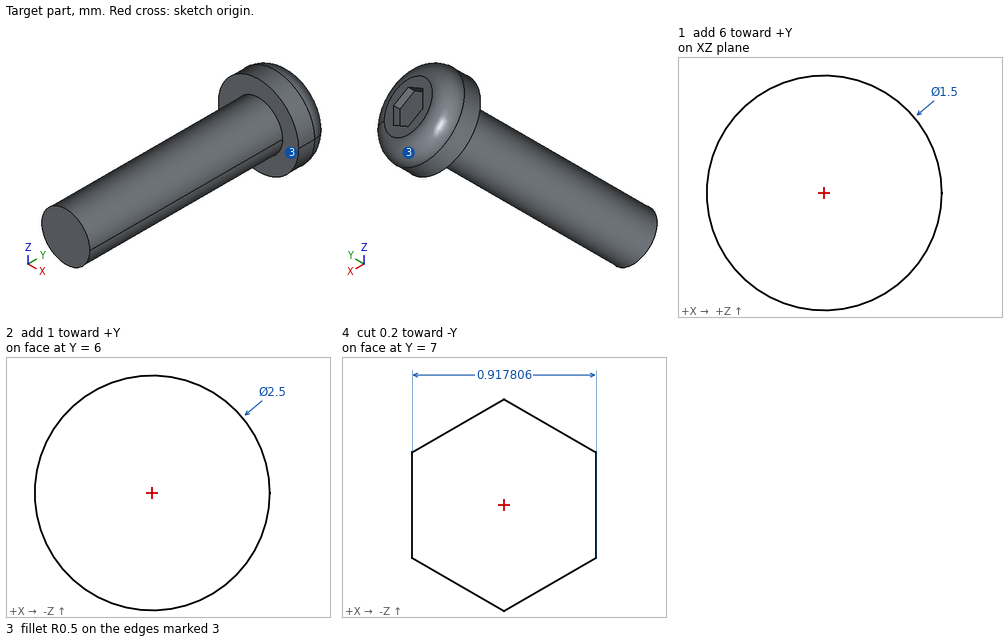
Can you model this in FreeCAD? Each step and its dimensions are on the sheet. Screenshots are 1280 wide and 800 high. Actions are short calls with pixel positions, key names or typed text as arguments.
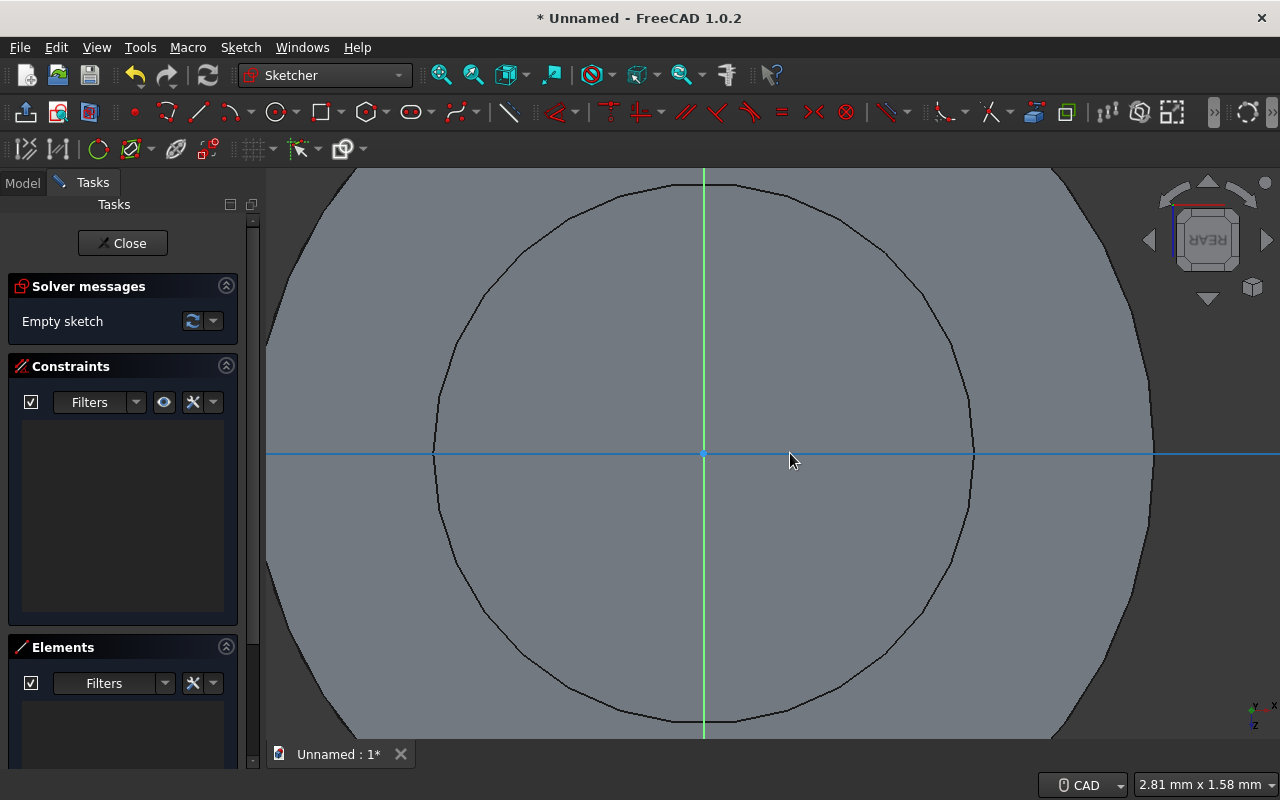
click(366, 112)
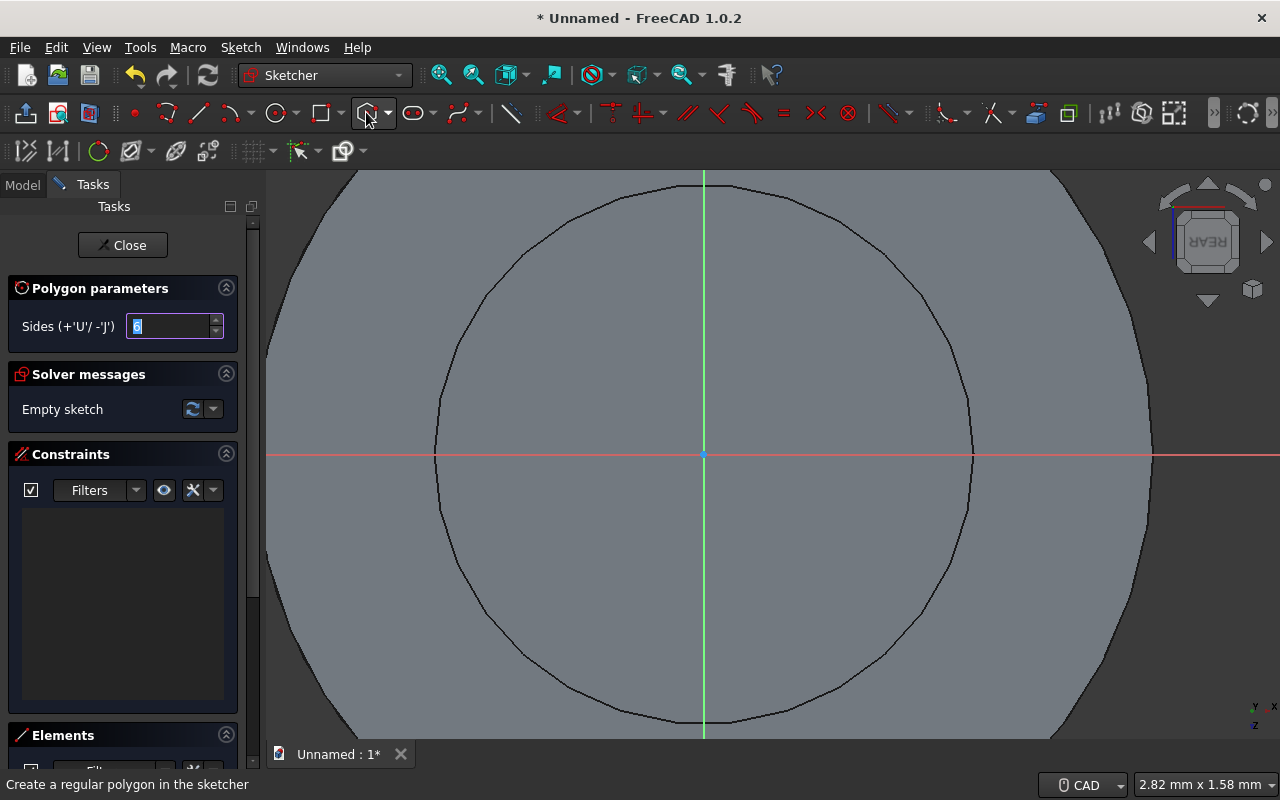
click(704, 454)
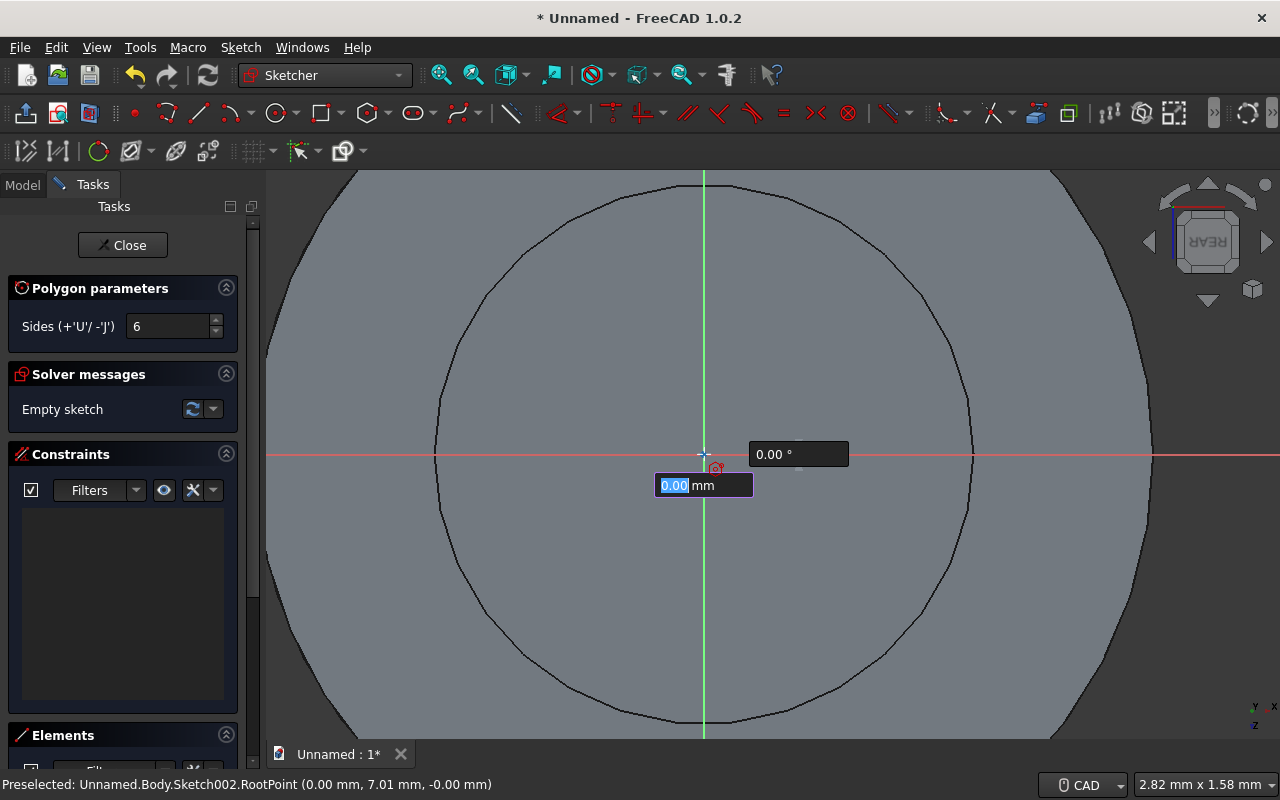
click(704, 264)
key(Escape)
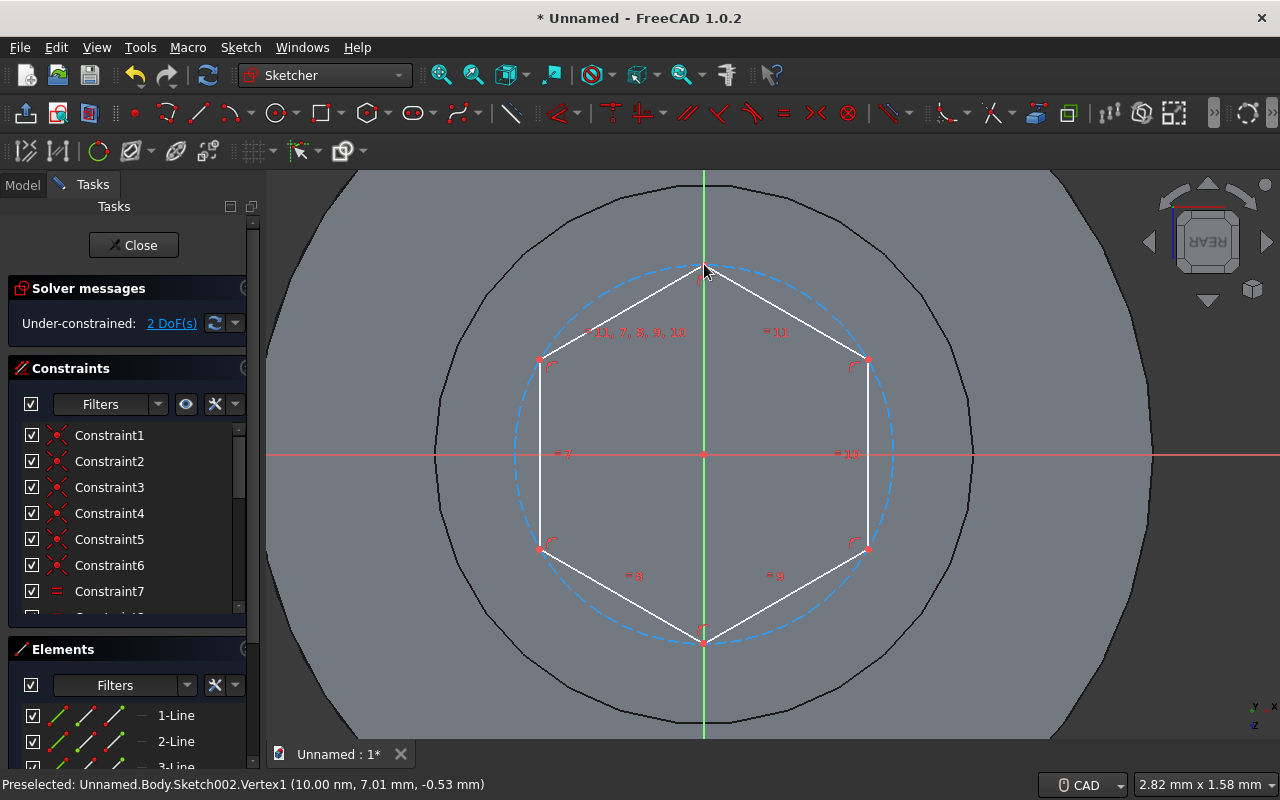
click(540, 417)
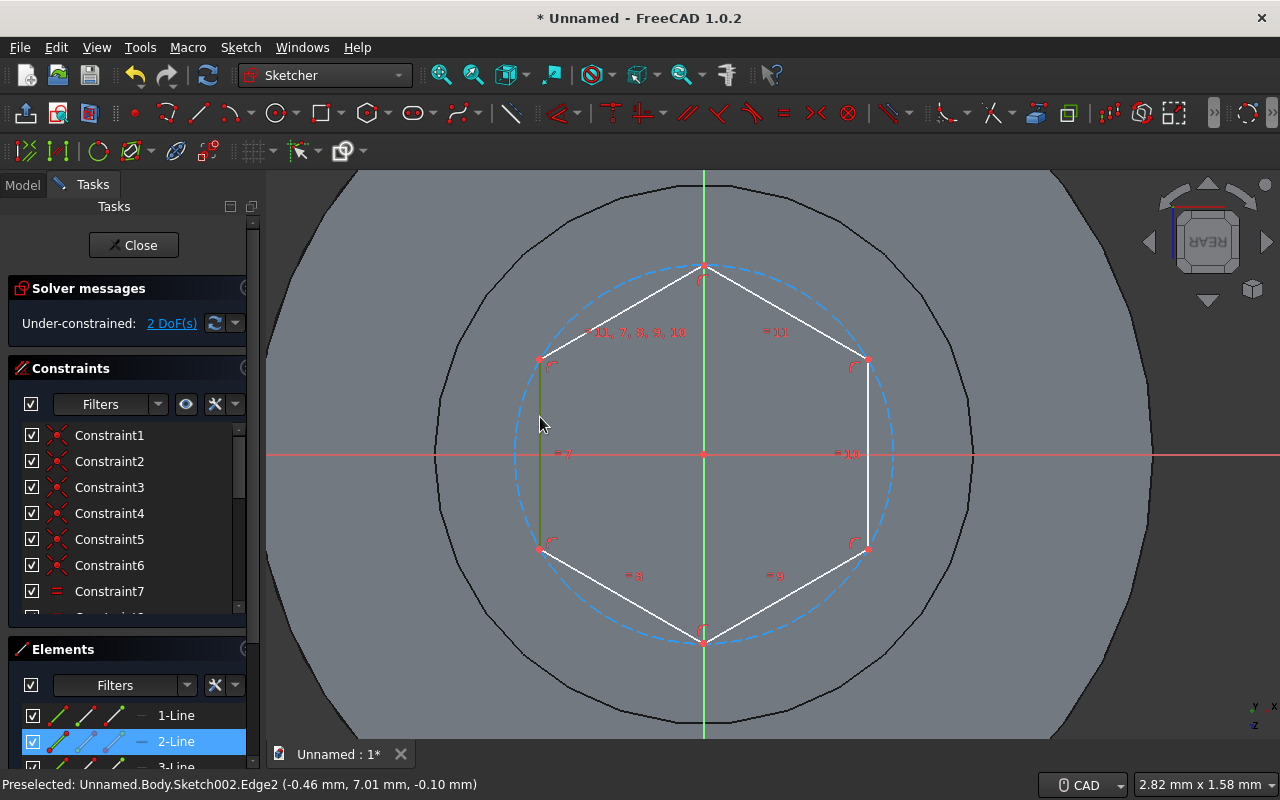
key(v)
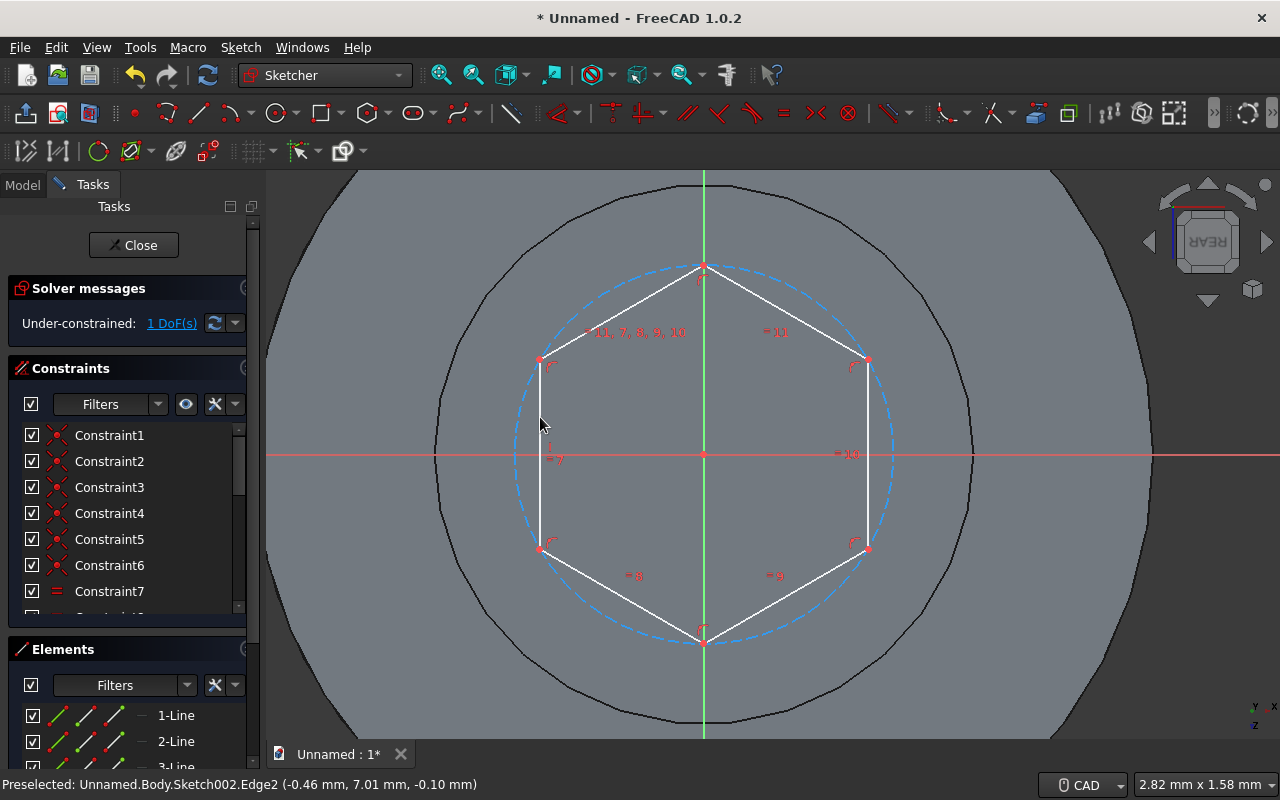
click(540, 360)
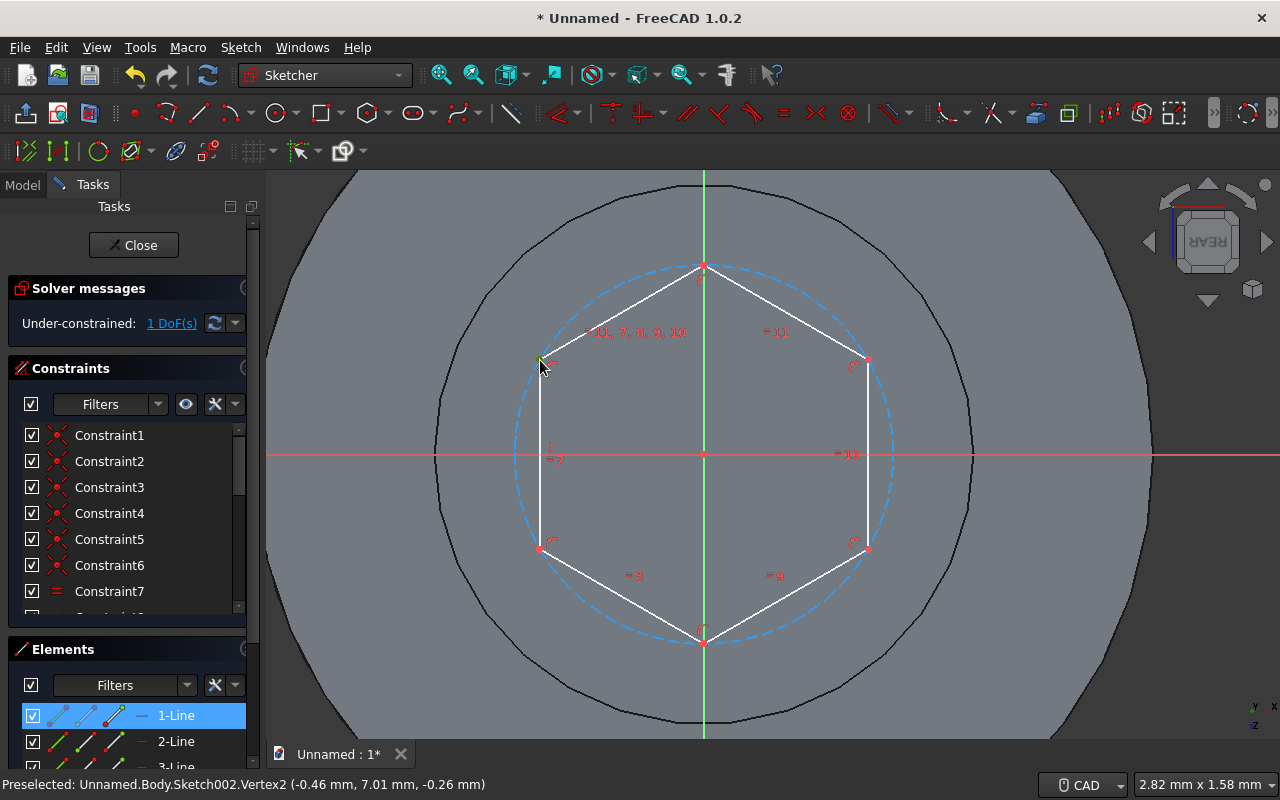
click(868, 549)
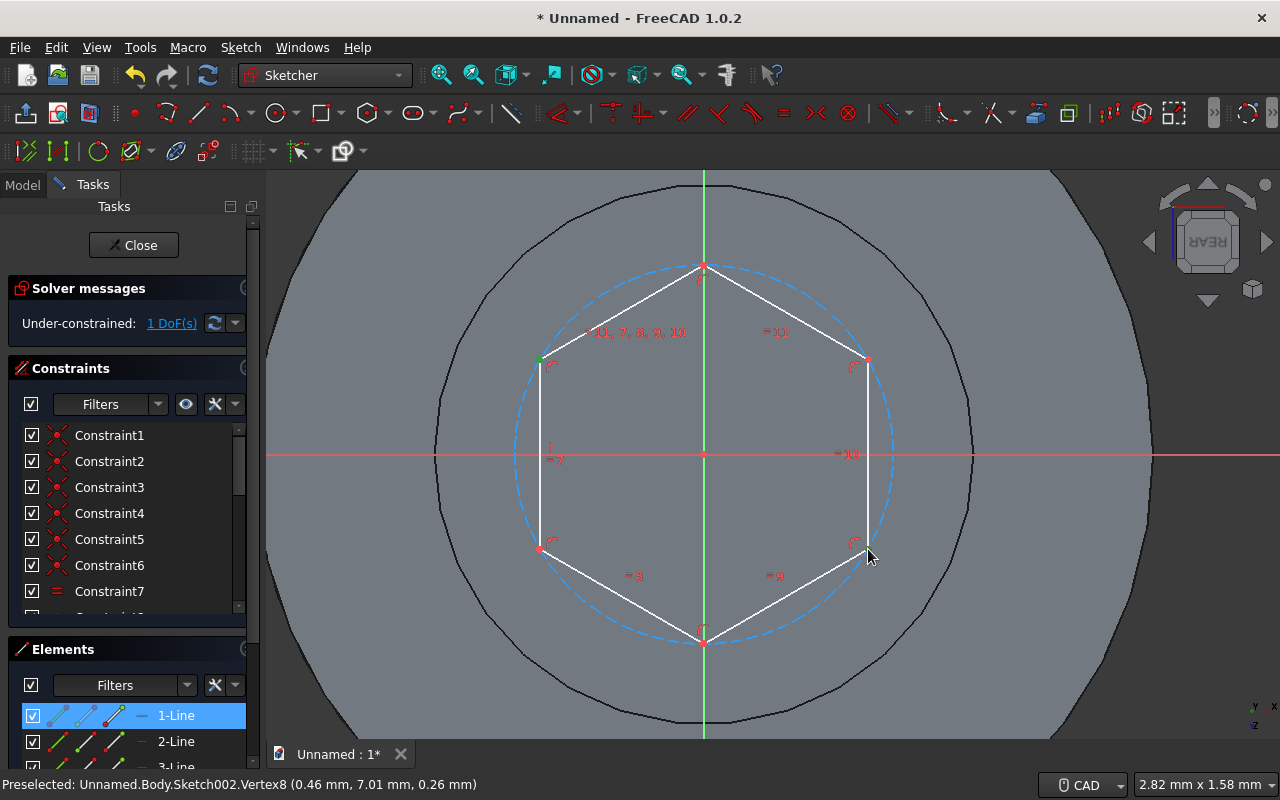
key(l)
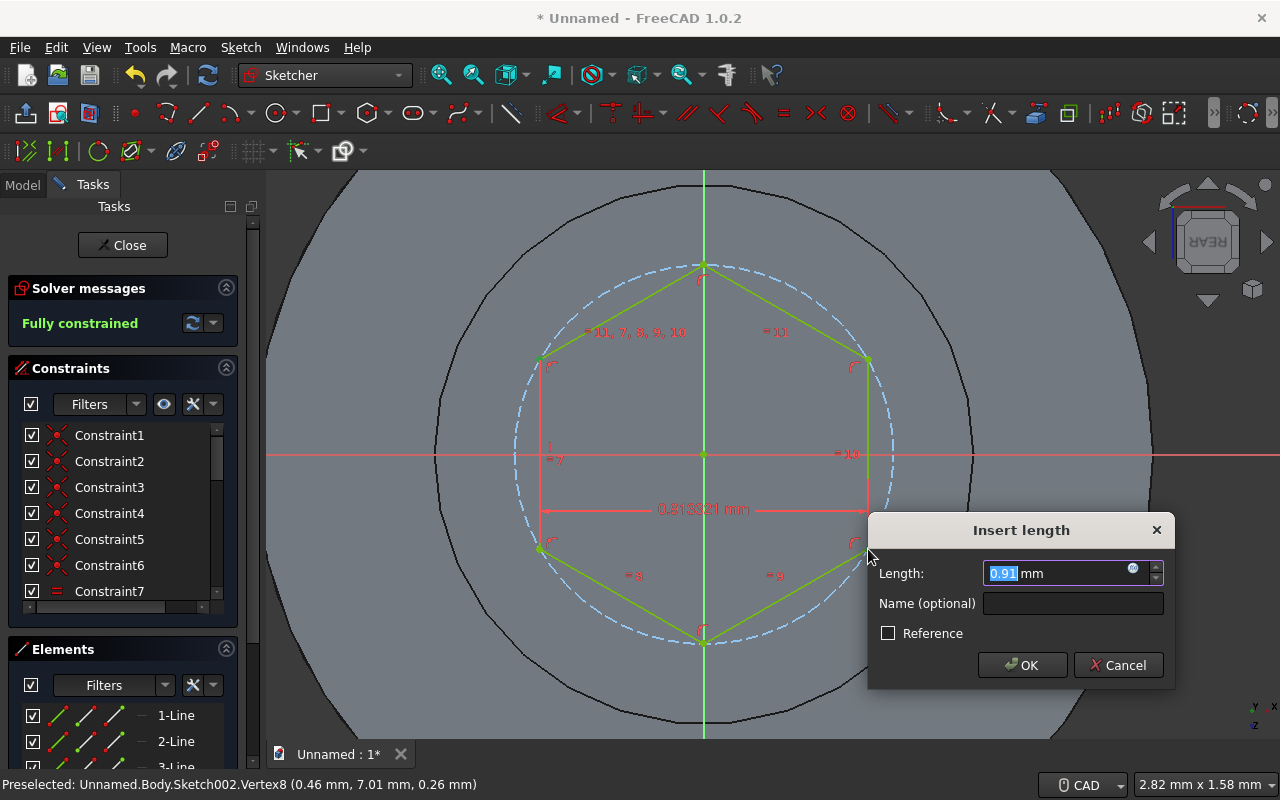
text(0.917806)
key(Return)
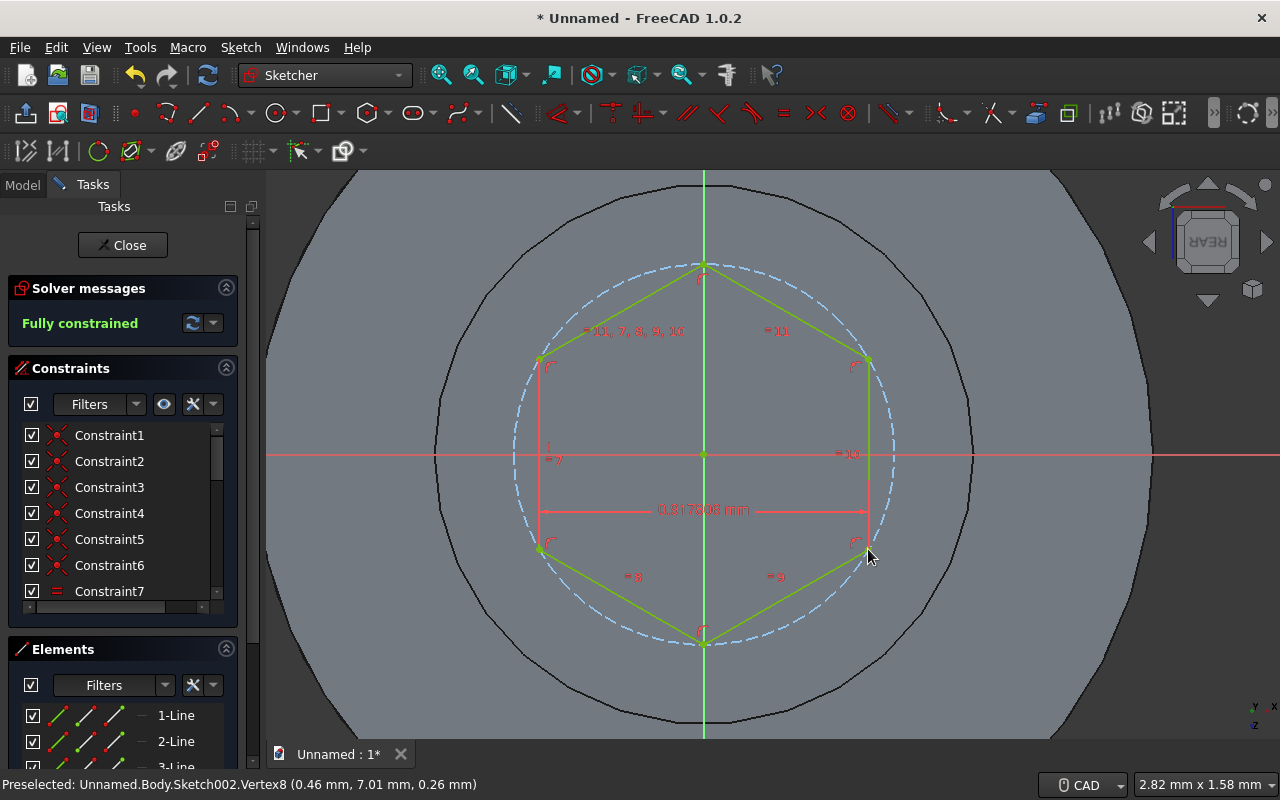
click(123, 245)